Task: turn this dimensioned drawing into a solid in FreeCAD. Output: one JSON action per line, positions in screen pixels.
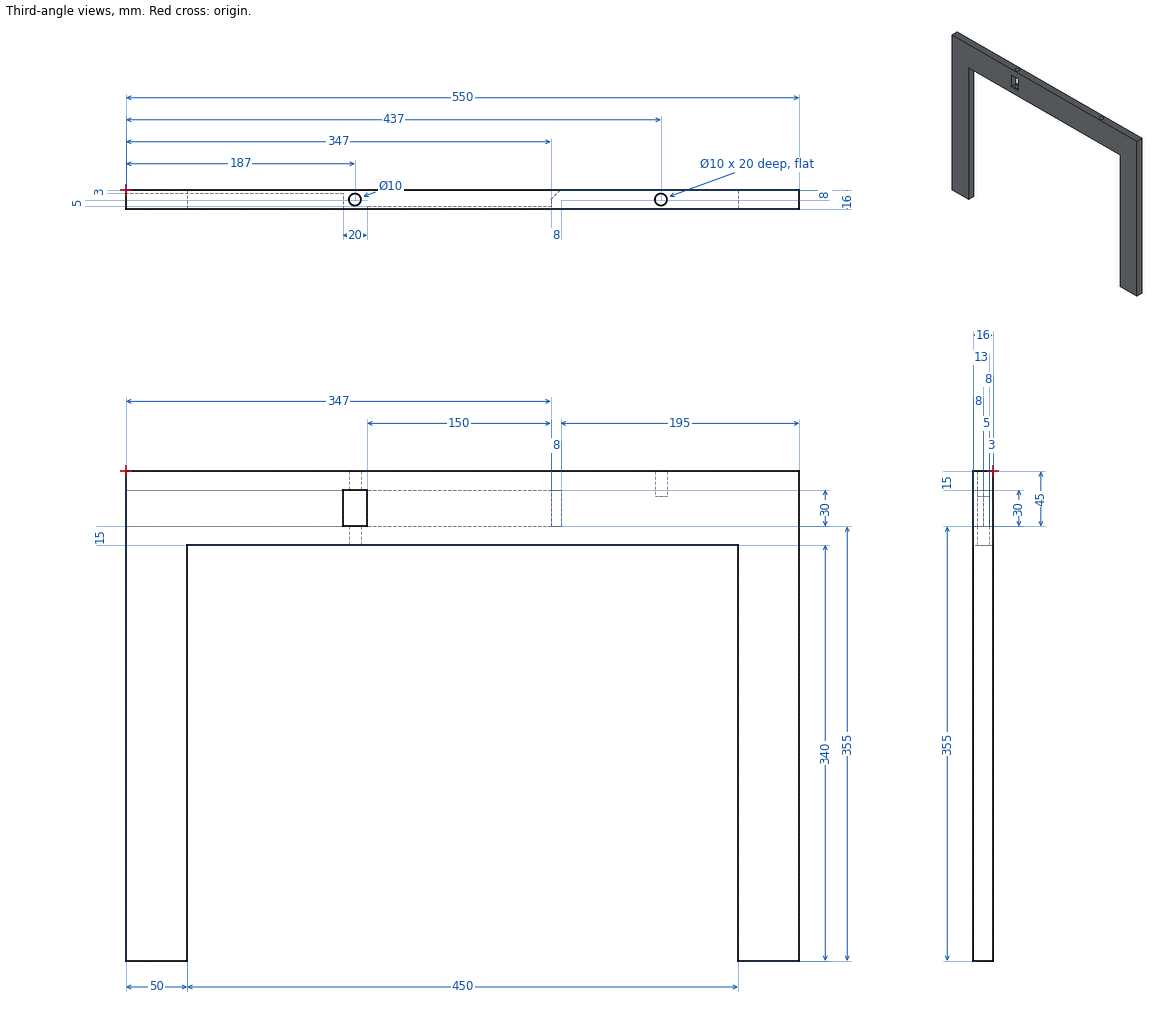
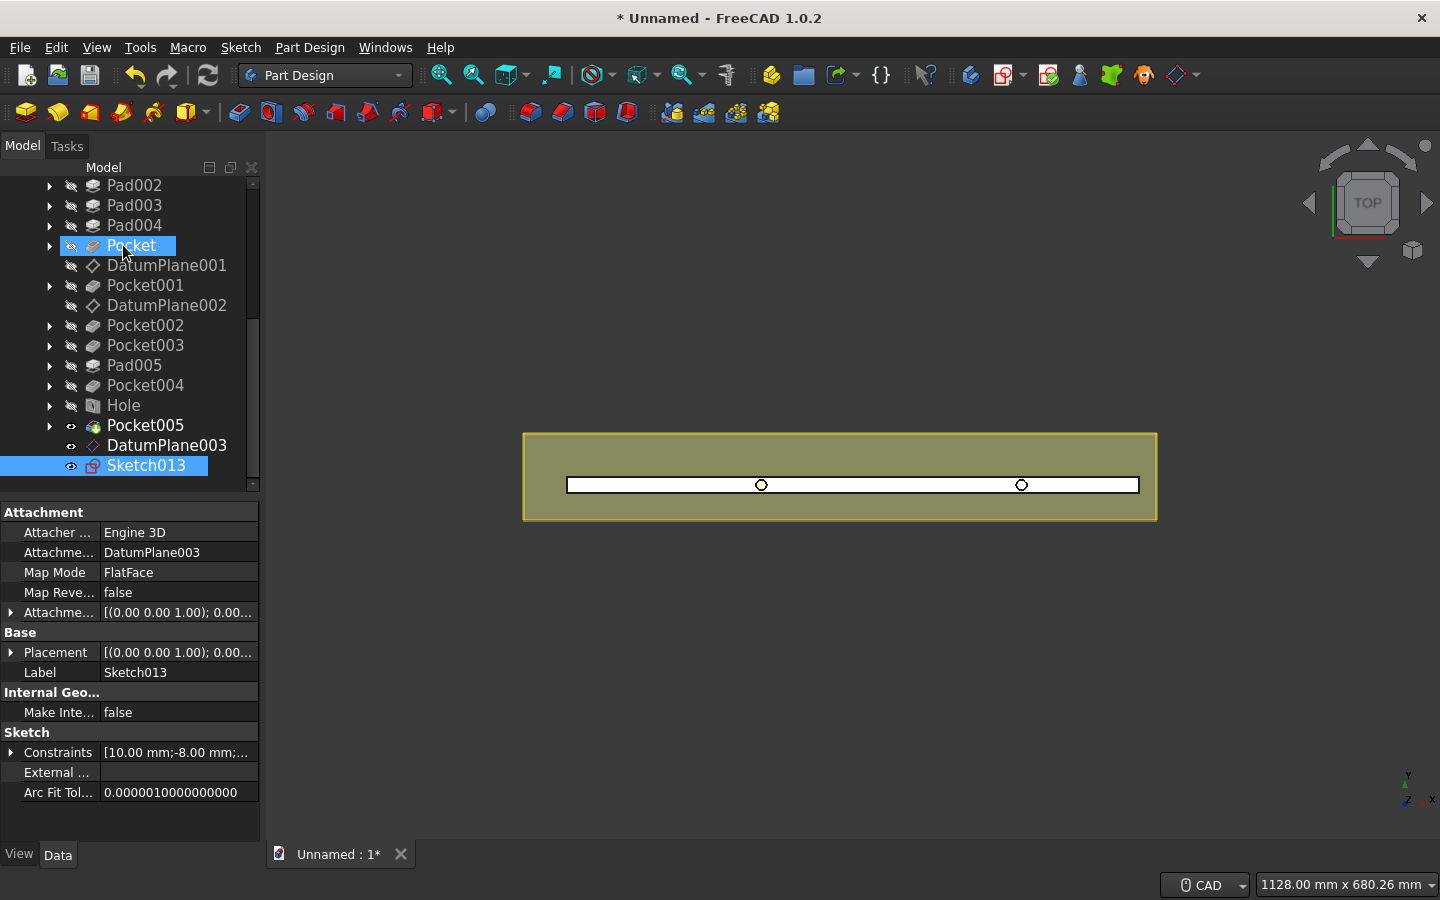
{"action": "left_click", "coordinate": [240, 112]}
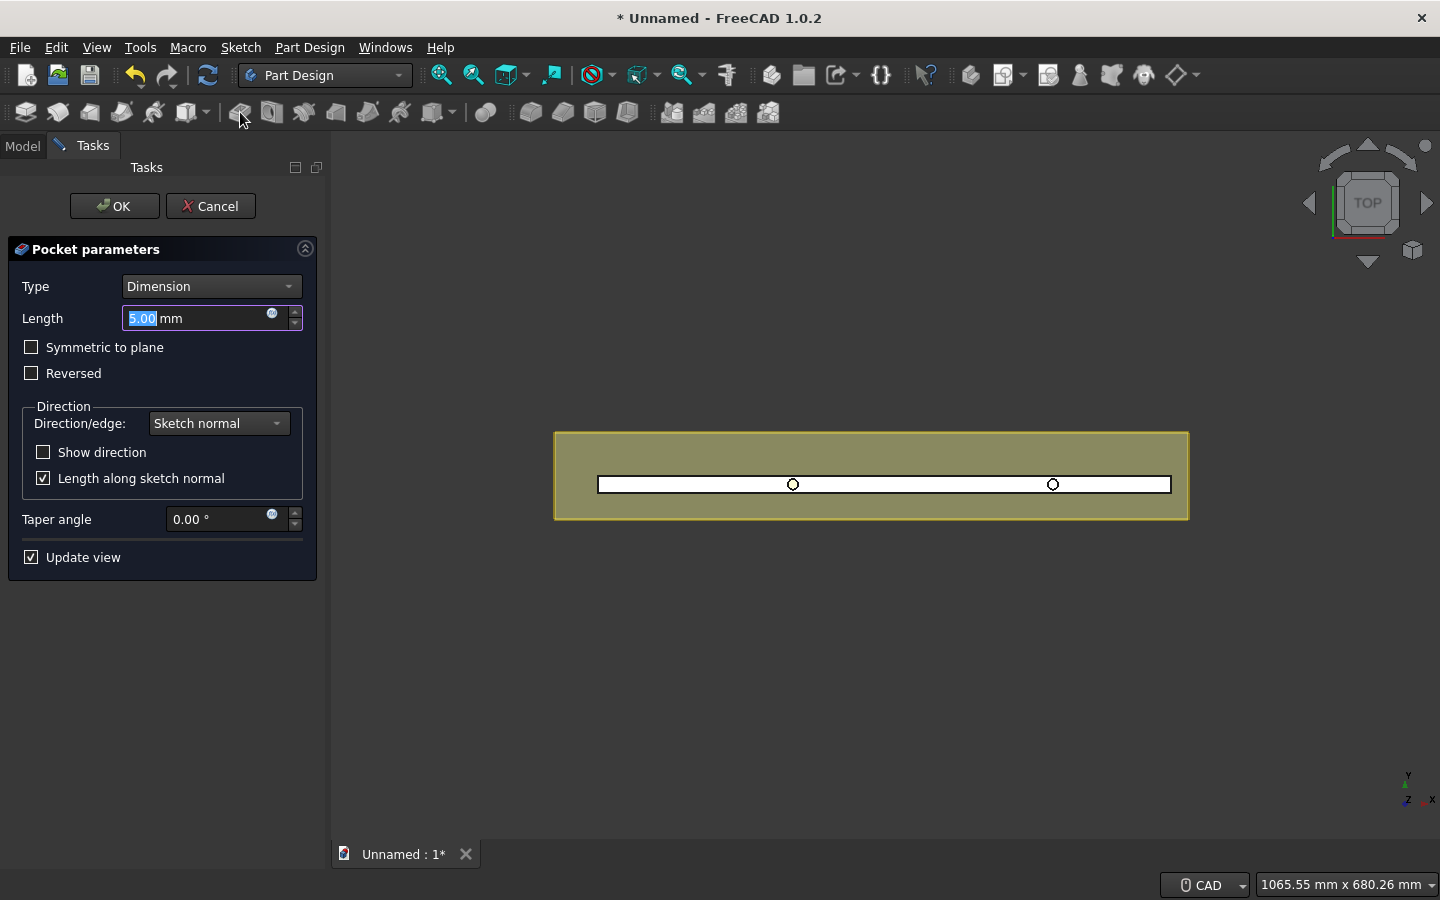
{"action": "type", "text": "355"}
{"action": "key", "text": "Tab"}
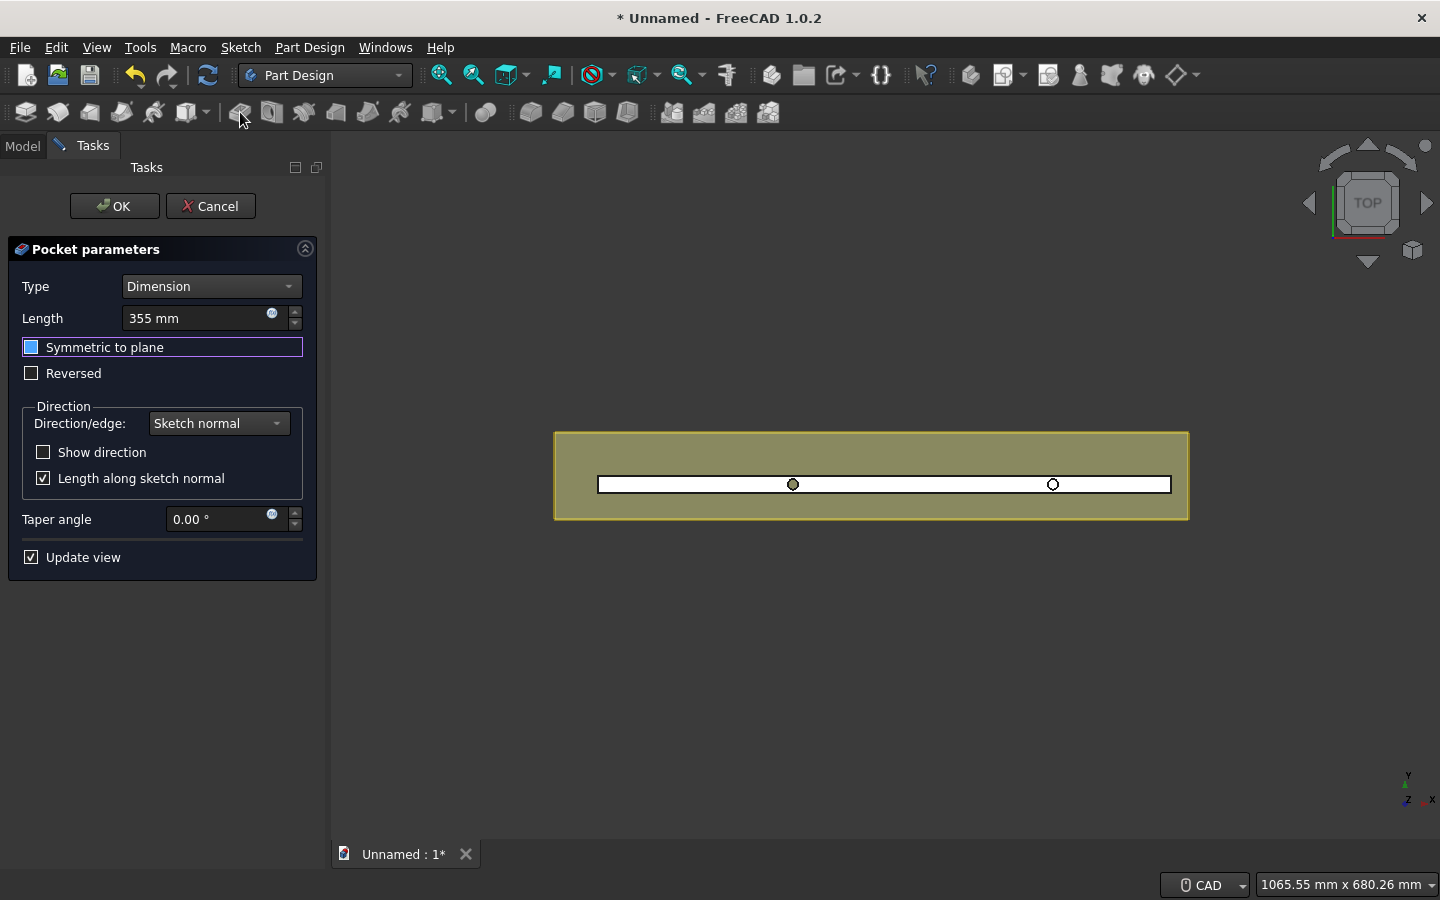
{"action": "left_click", "coordinate": [115, 206]}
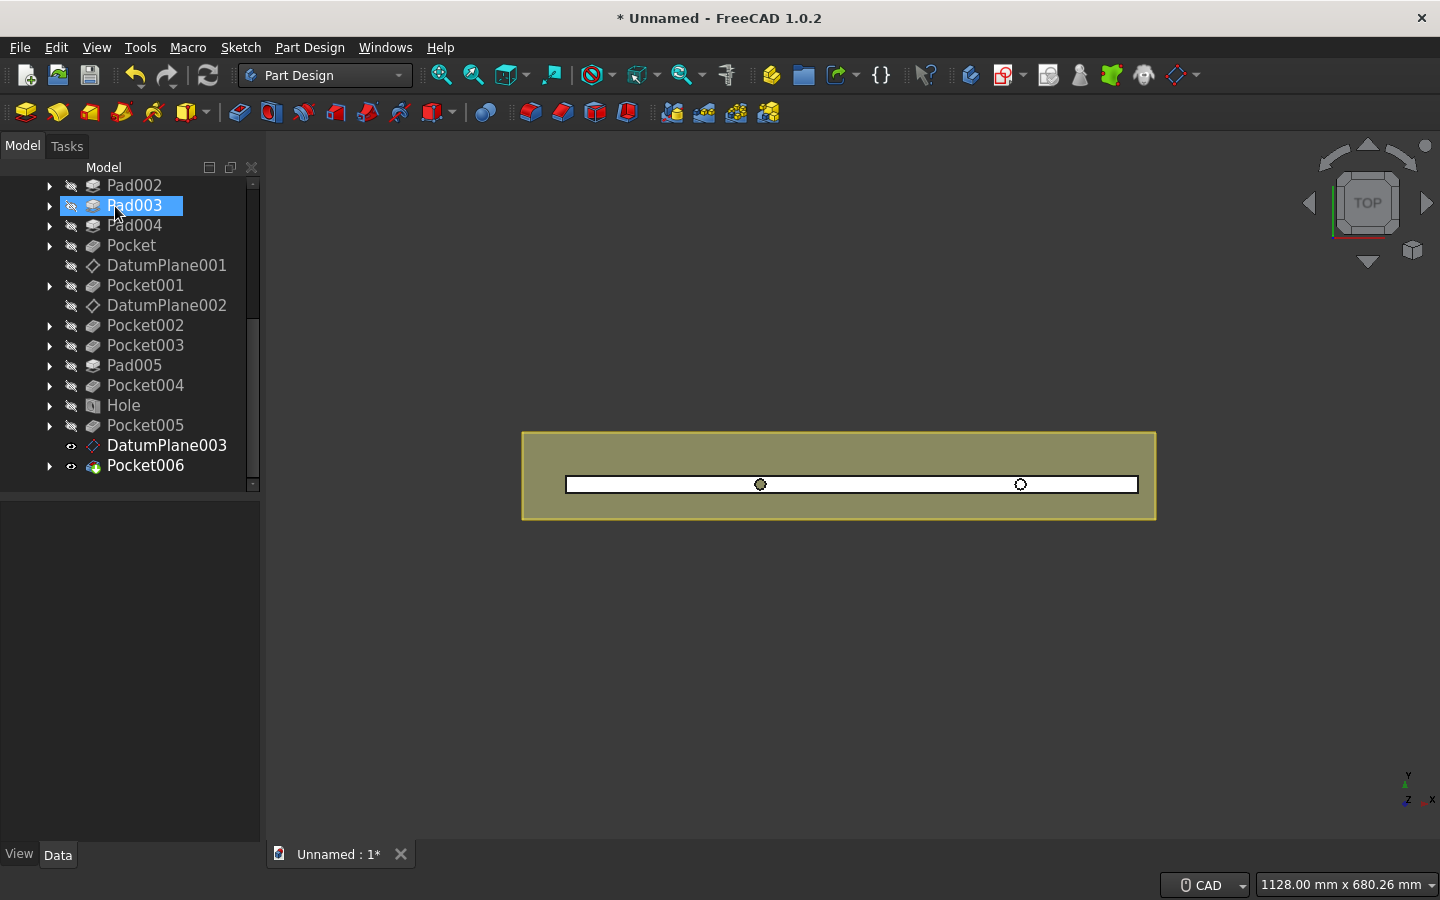
{"action": "left_click", "coordinate": [116, 446]}
{"action": "key", "text": "space"}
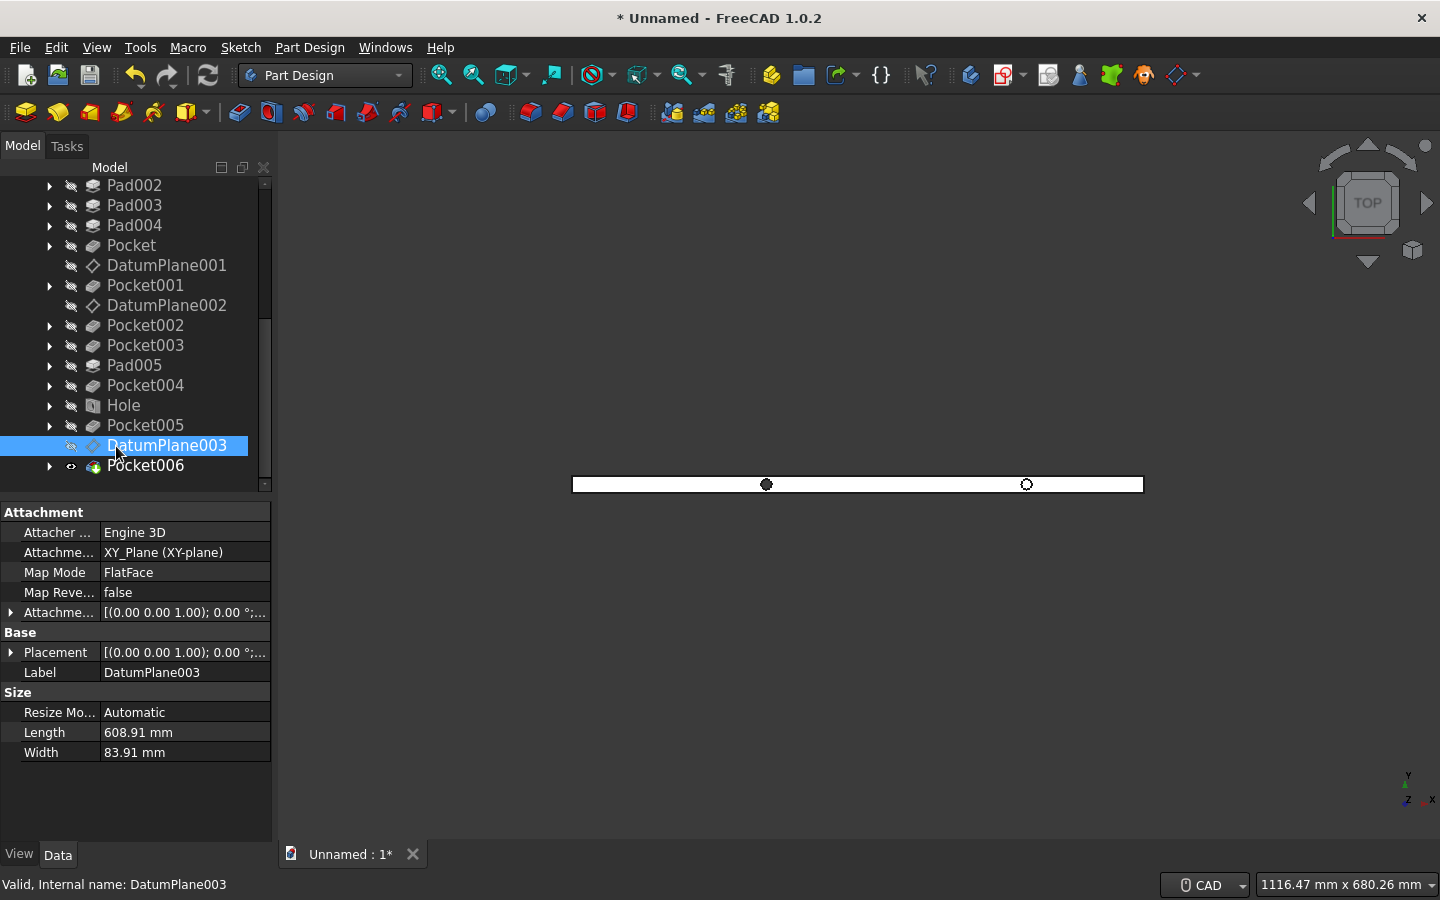
{"action": "key", "text": "0"}